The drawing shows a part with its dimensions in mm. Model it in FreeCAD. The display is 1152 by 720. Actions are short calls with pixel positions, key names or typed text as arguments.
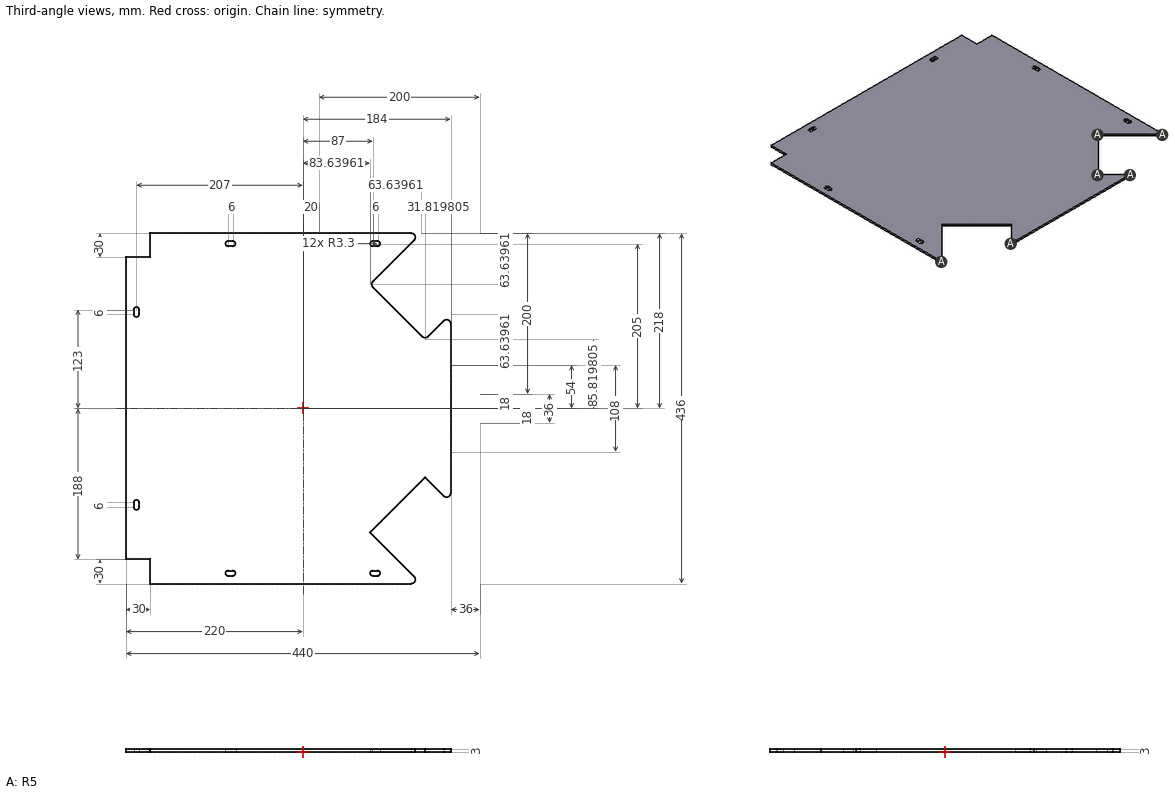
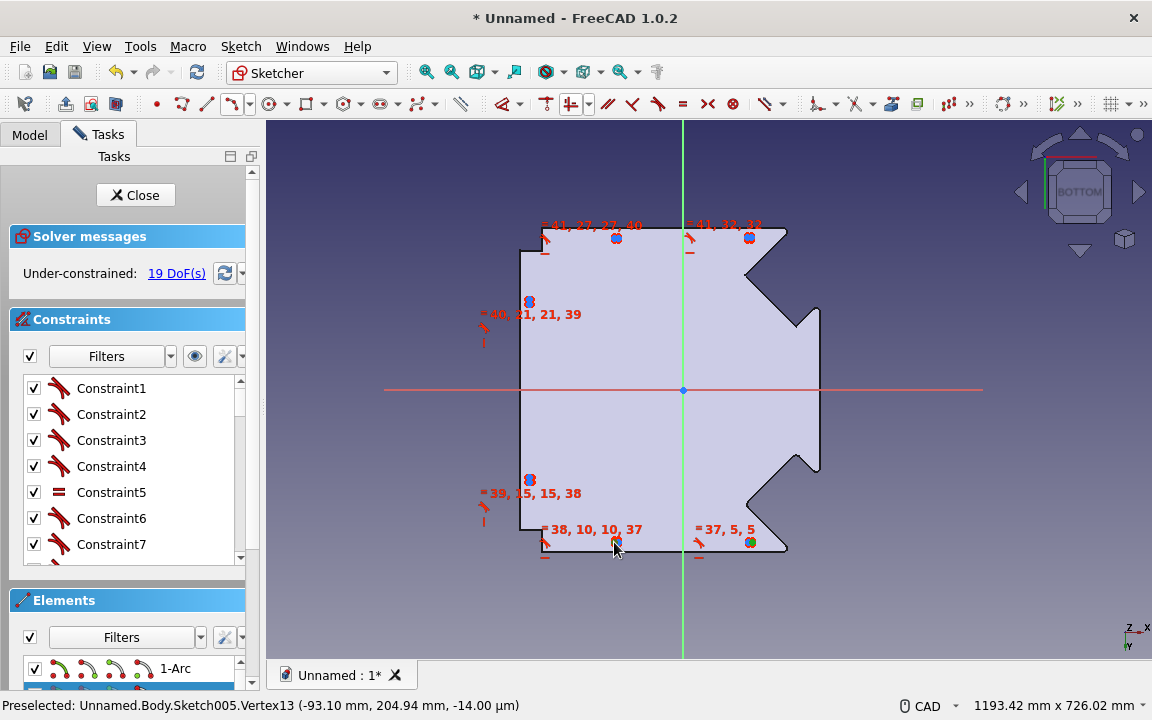
click(683, 596)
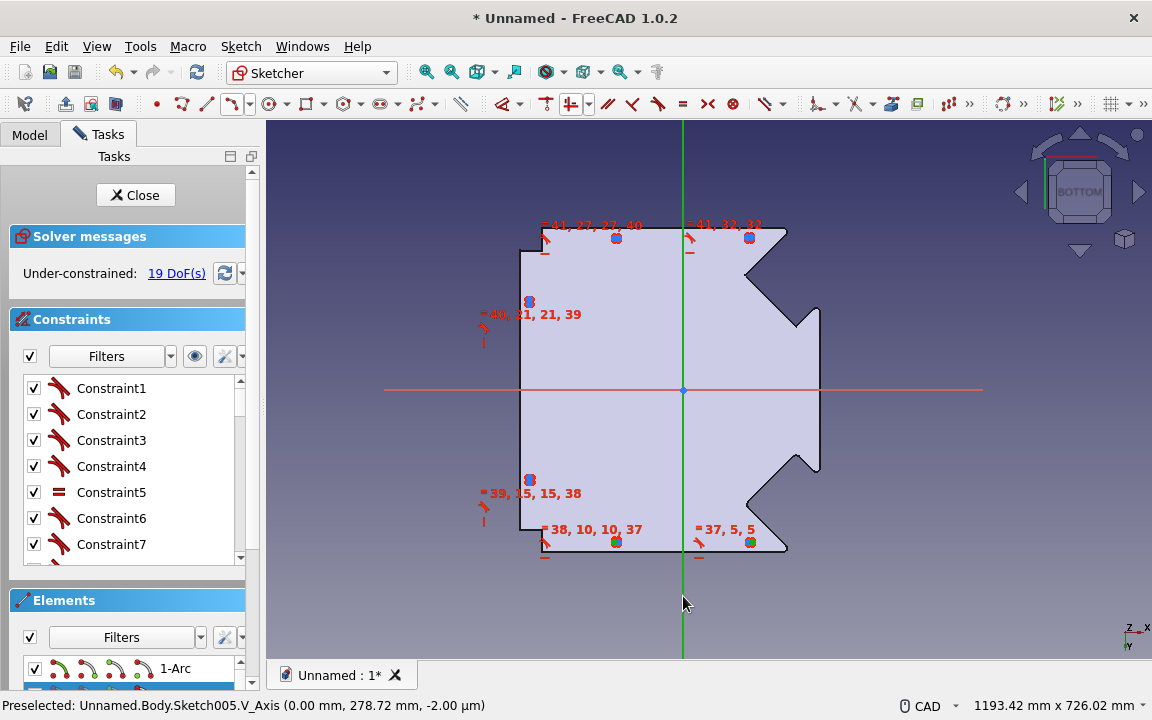
key(s)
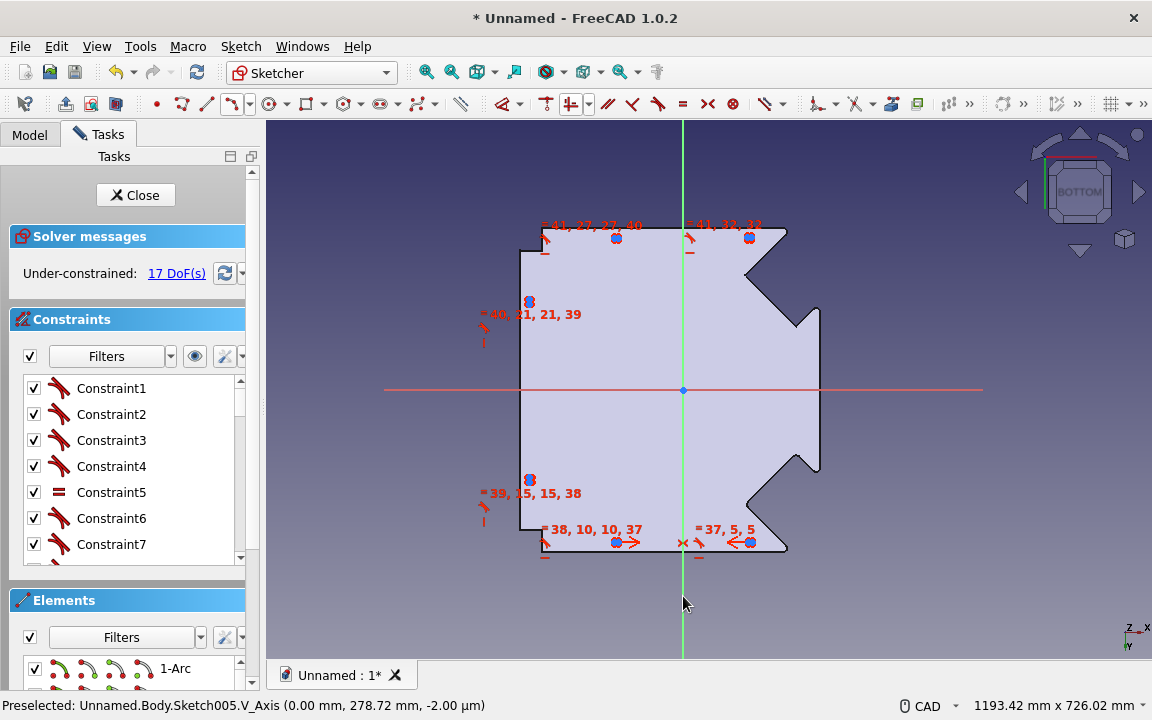
scroll(530, 477, up, 9)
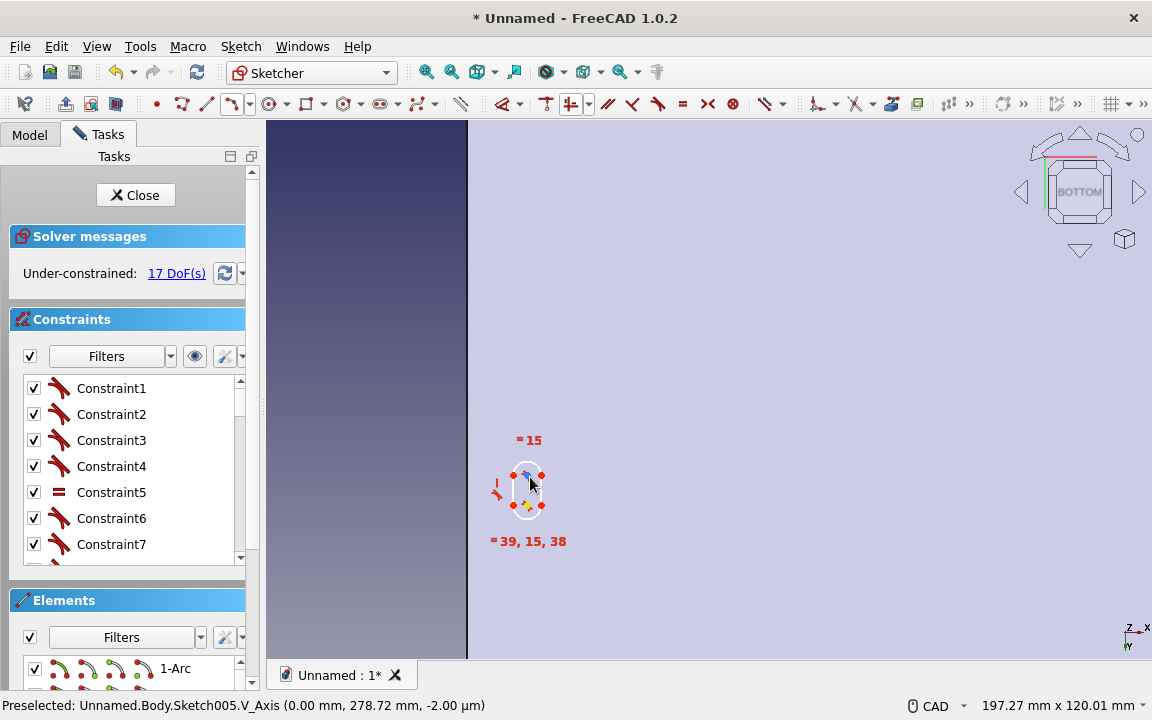
click(527, 475)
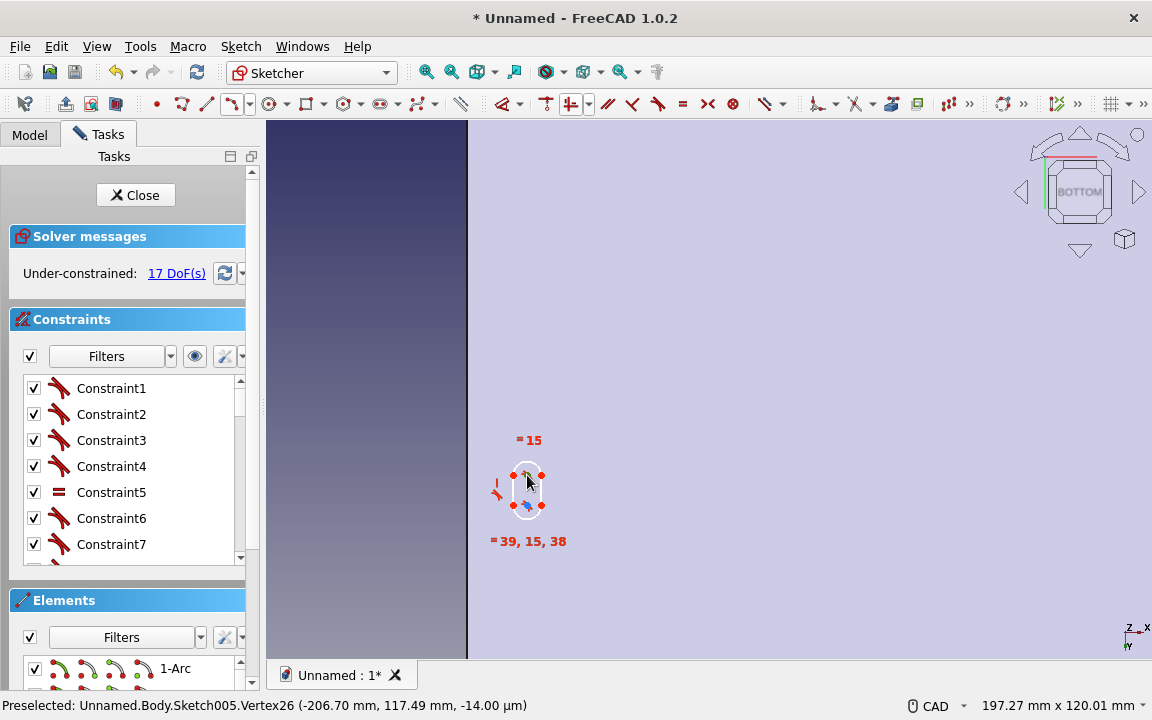
scroll(530, 477, down, 9)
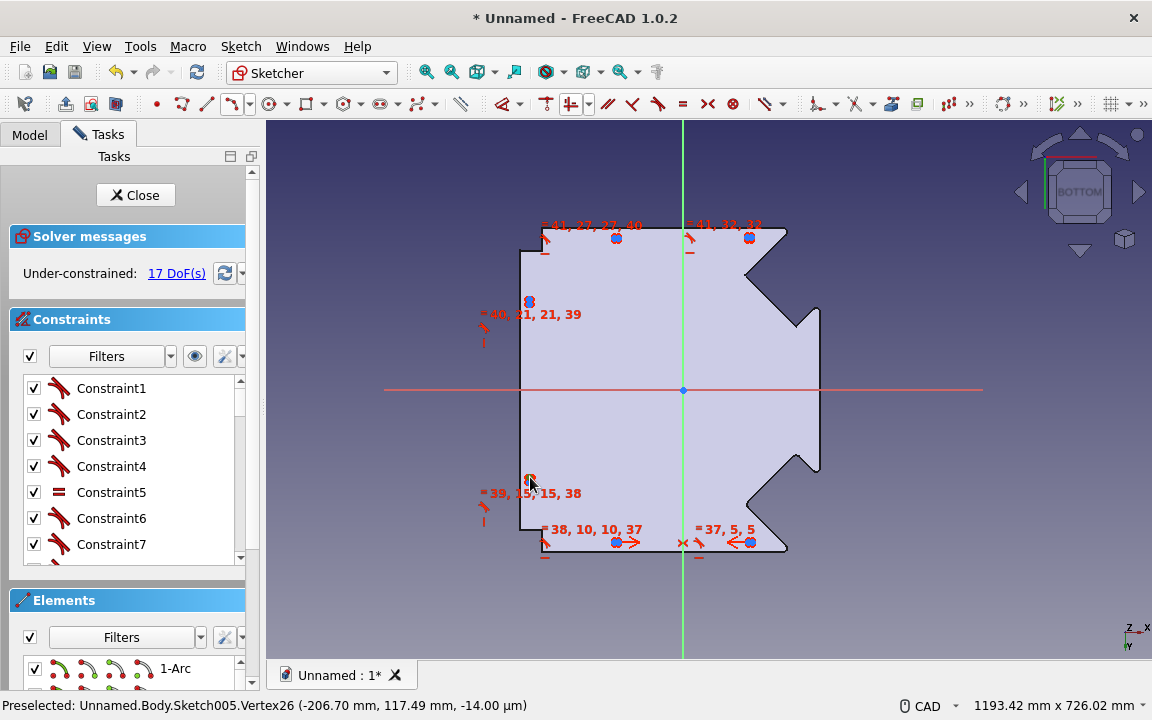
scroll(529, 304, up, 9)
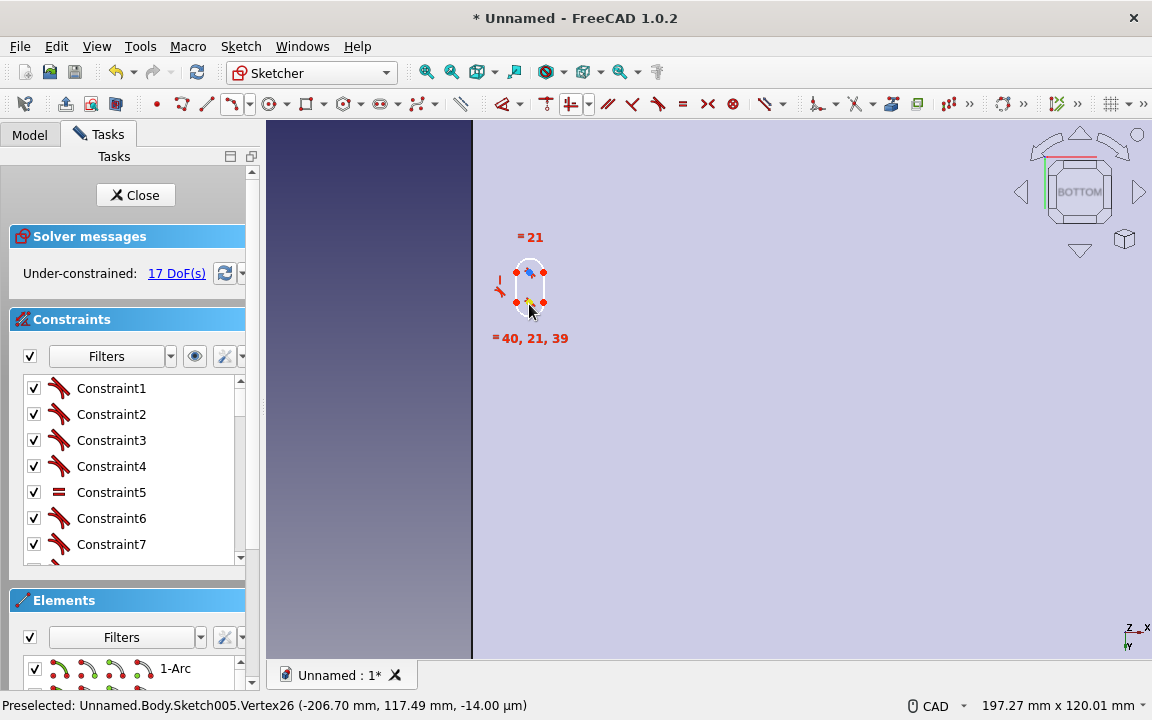
click(530, 303)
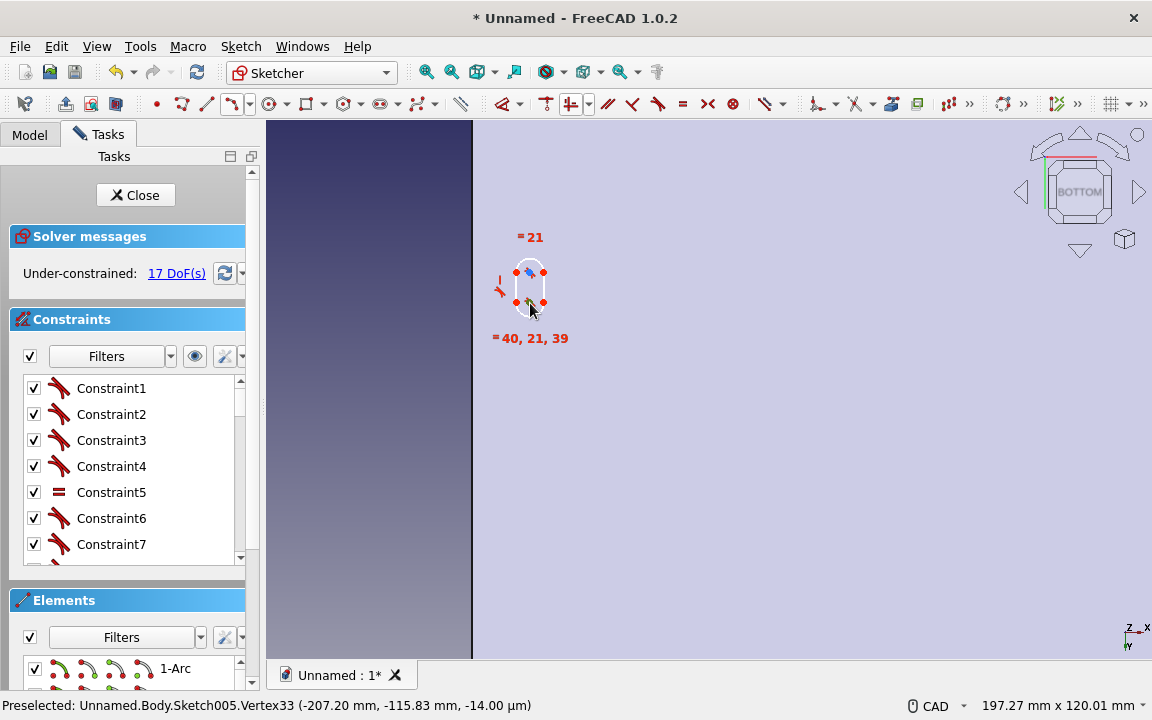
scroll(529, 304, down, 9)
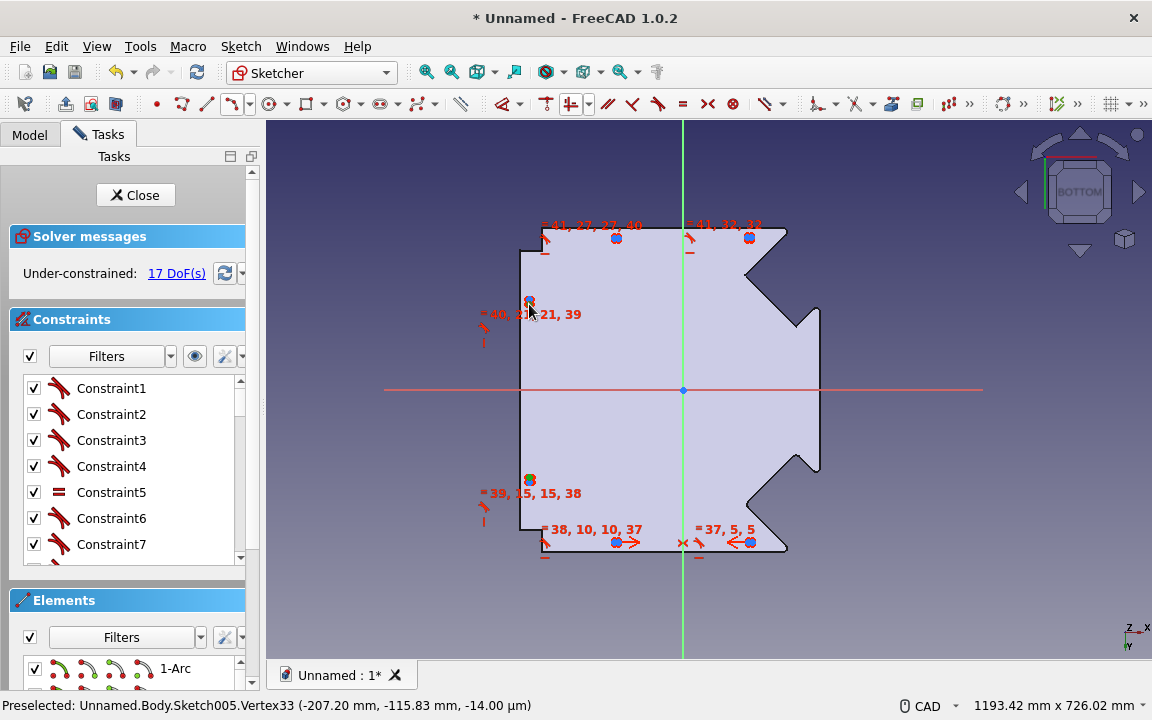
click(393, 390)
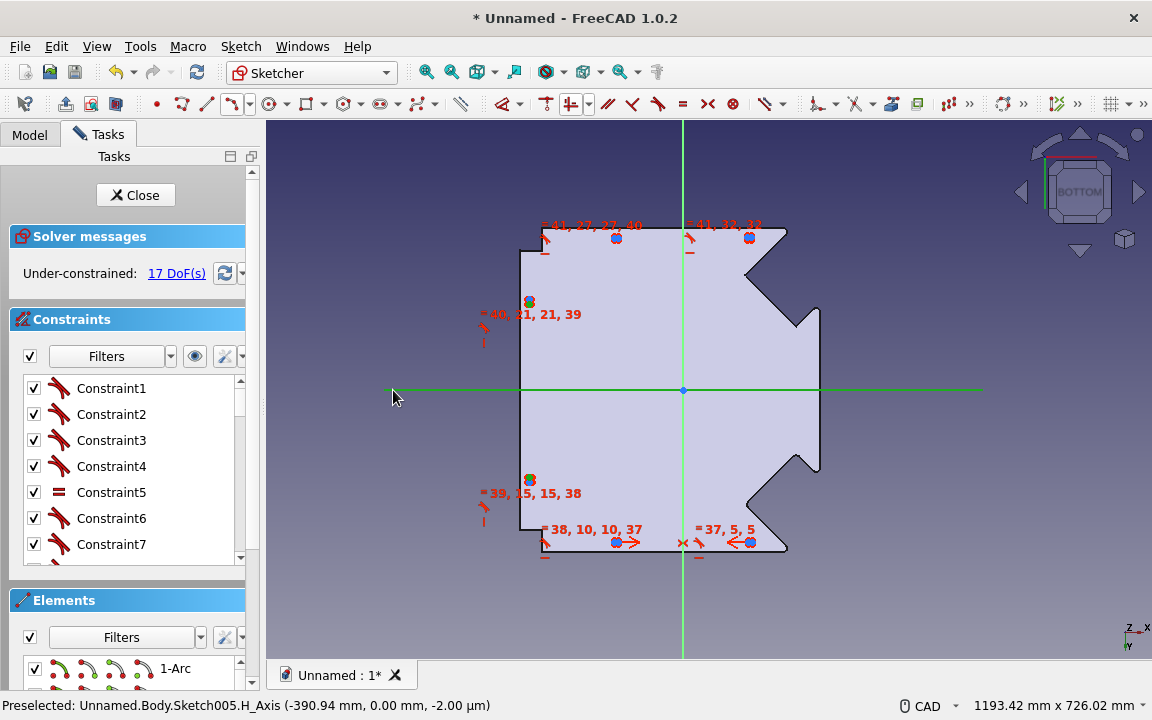
key(s)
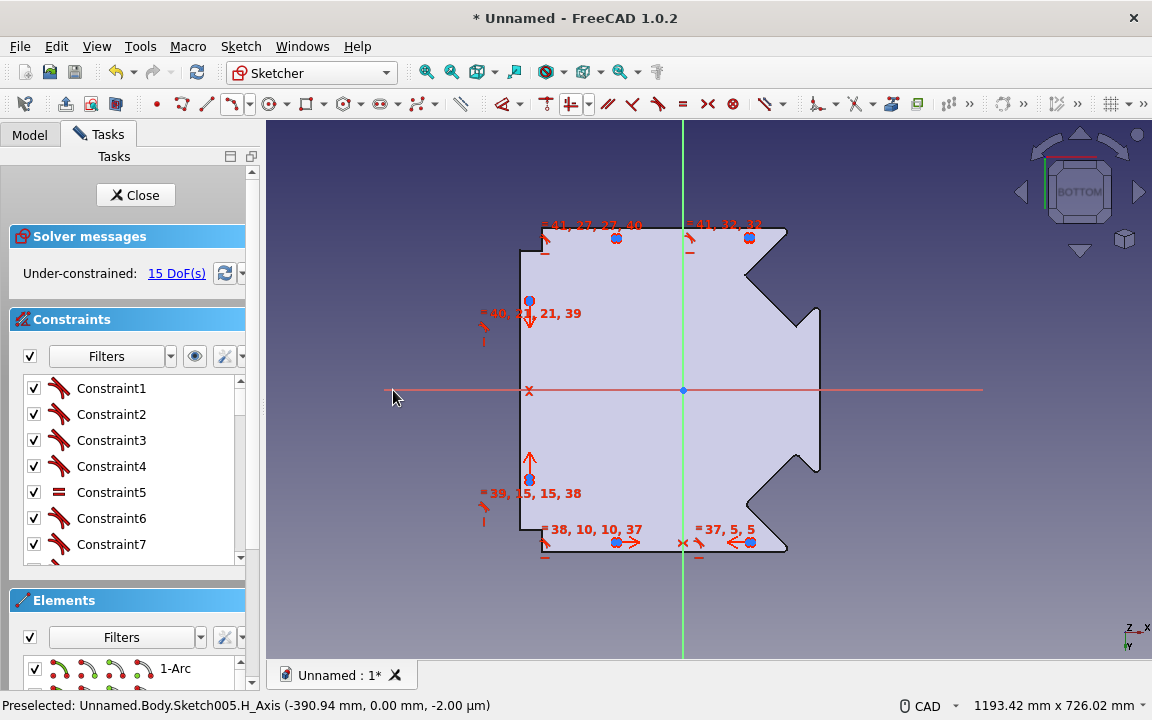
scroll(614, 542, up, 9)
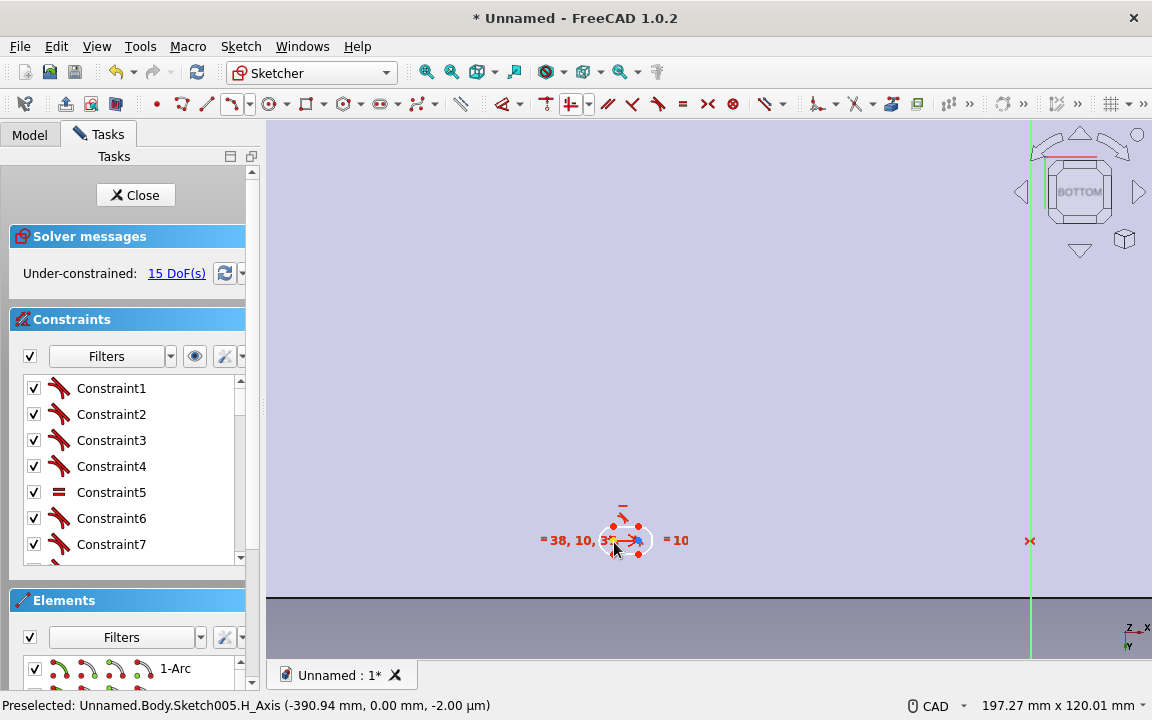
click(613, 541)